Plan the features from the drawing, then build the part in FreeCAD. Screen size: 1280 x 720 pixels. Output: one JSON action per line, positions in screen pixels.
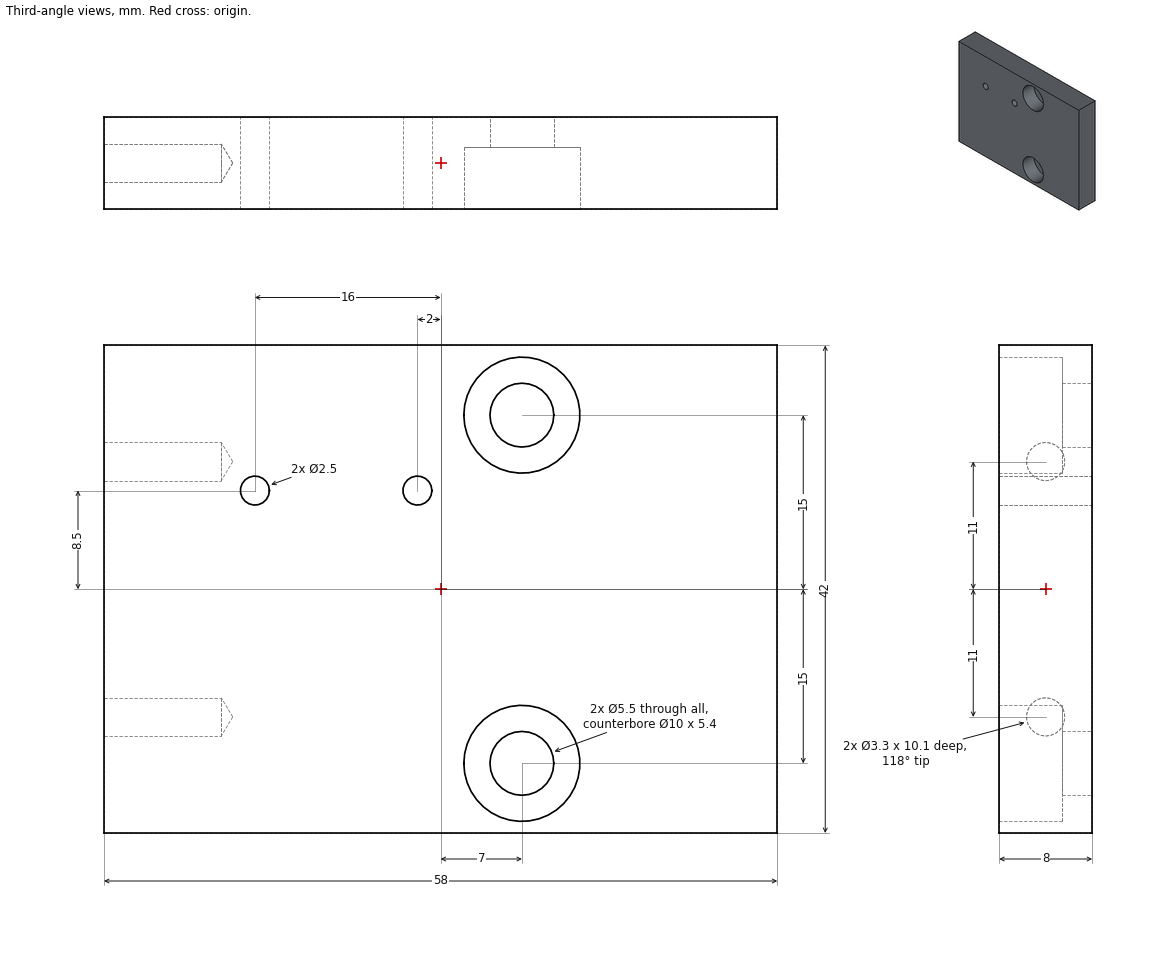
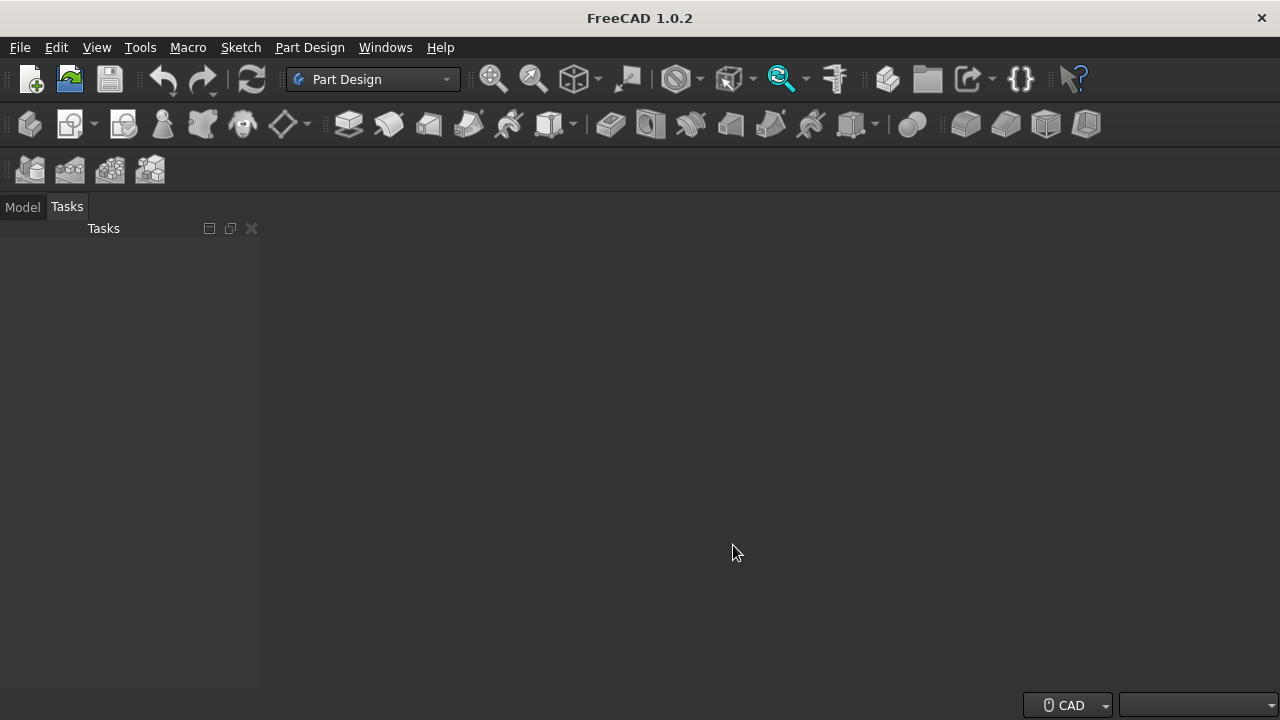
{"action": "left_click", "coordinate": [30, 80]}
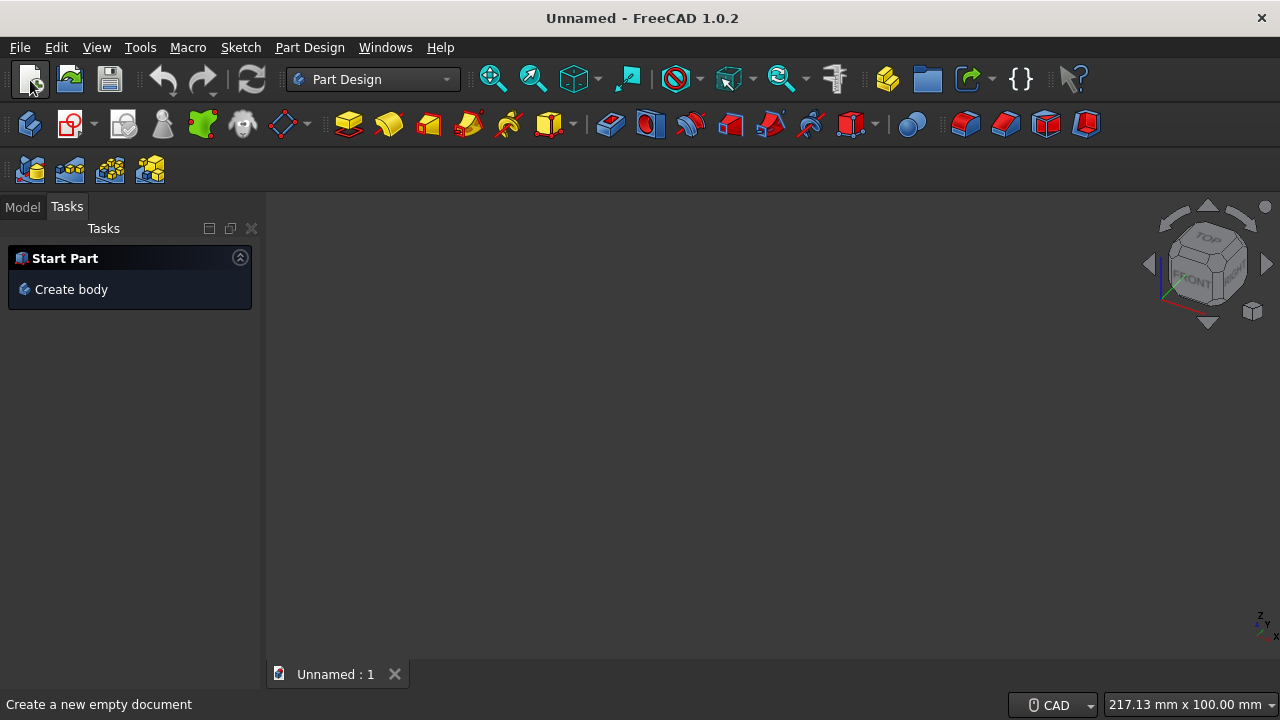
{"action": "left_click", "coordinate": [70, 124]}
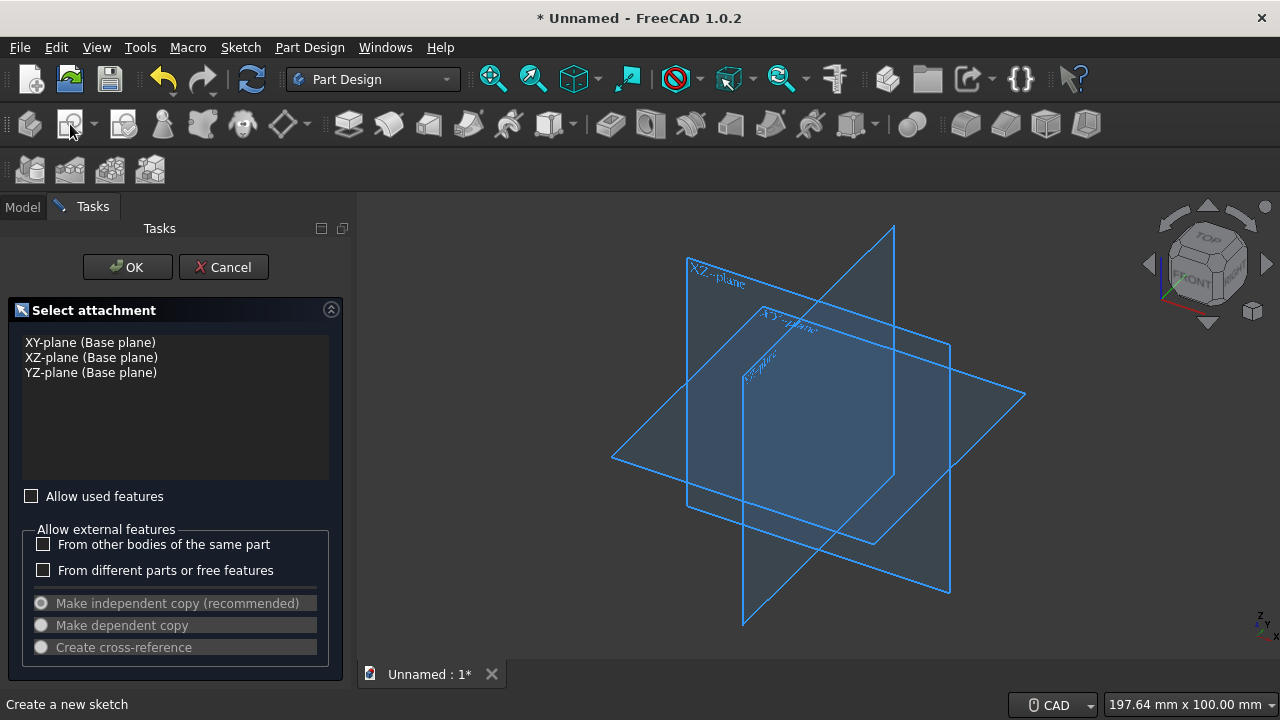
{"action": "left_click", "coordinate": [82, 358]}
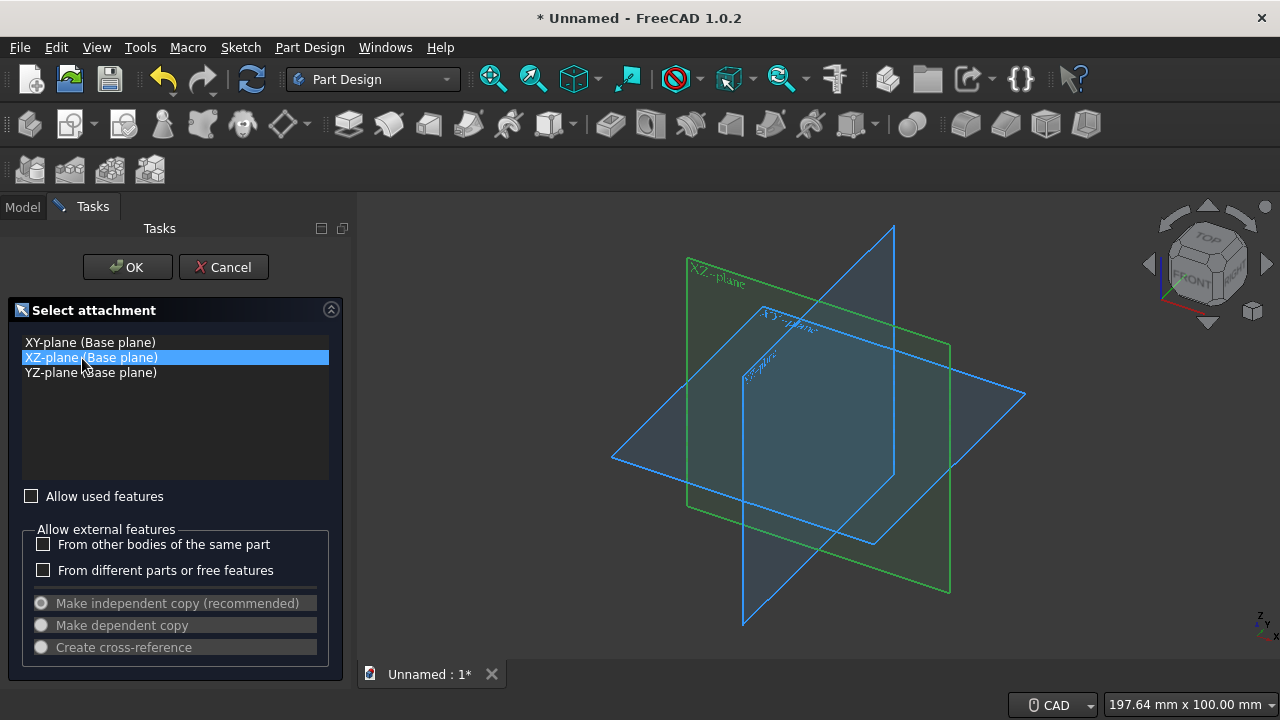
{"action": "left_click", "coordinate": [128, 267]}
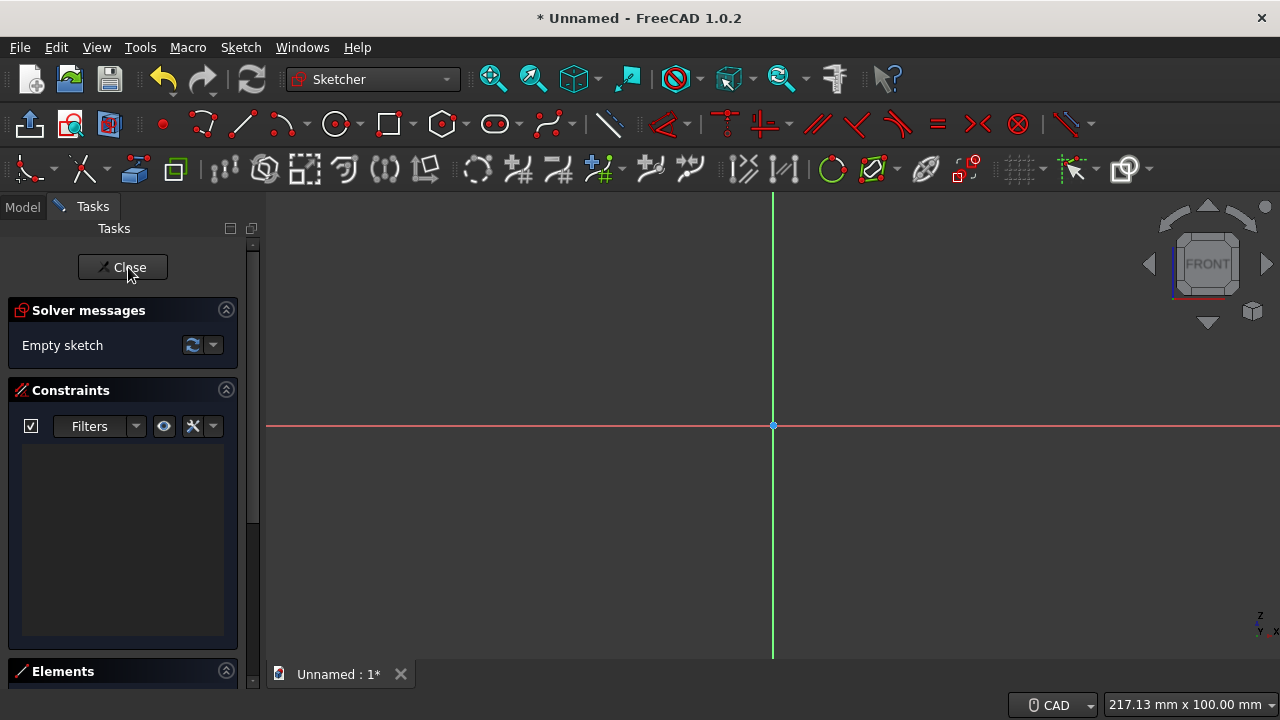
{"action": "scroll", "coordinate": [912, 425], "scroll_direction": "up", "scroll_amount": 2}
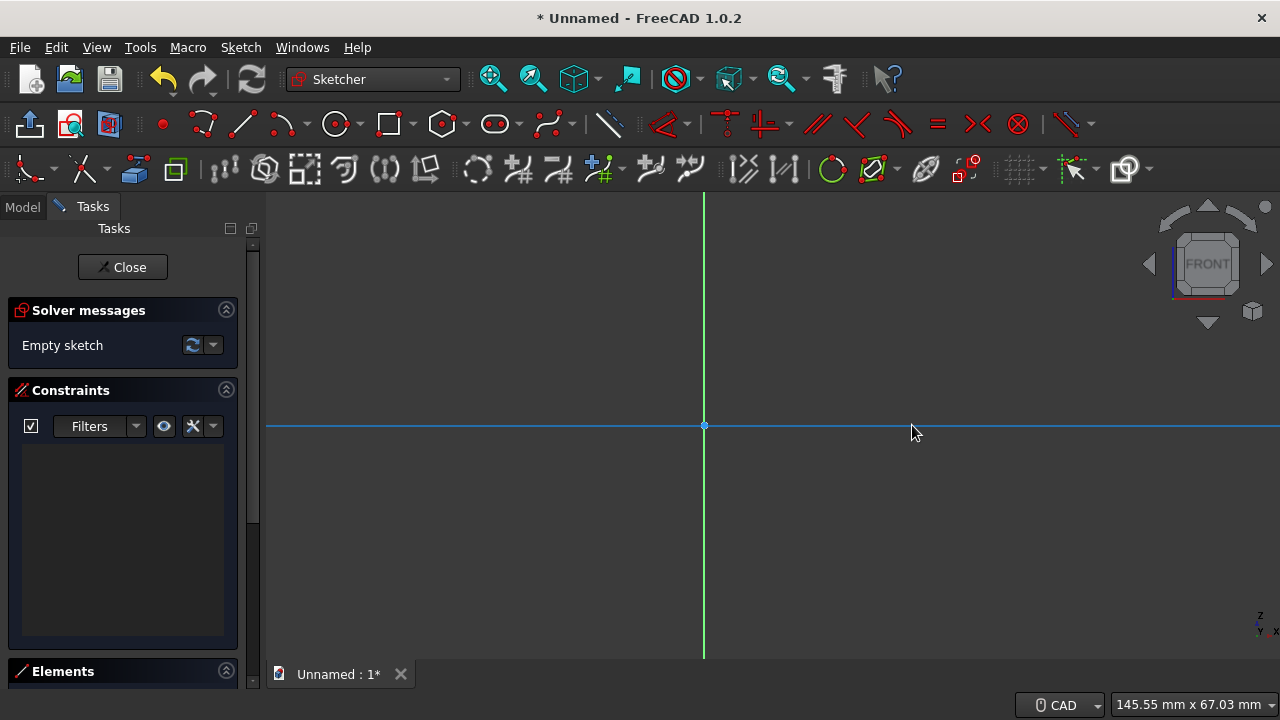
{"action": "key", "text": "g v"}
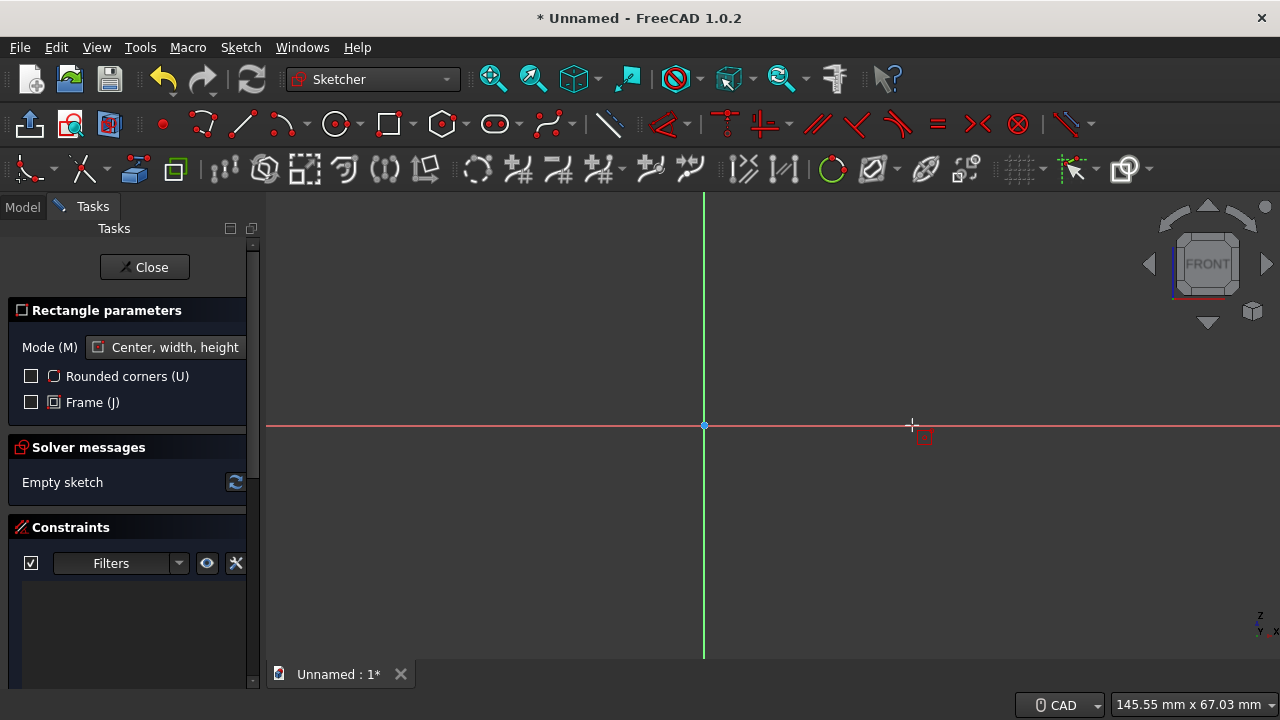
{"action": "left_click", "coordinate": [704, 426]}
{"action": "left_click", "coordinate": [906, 279]}
{"action": "key", "text": "Escape"}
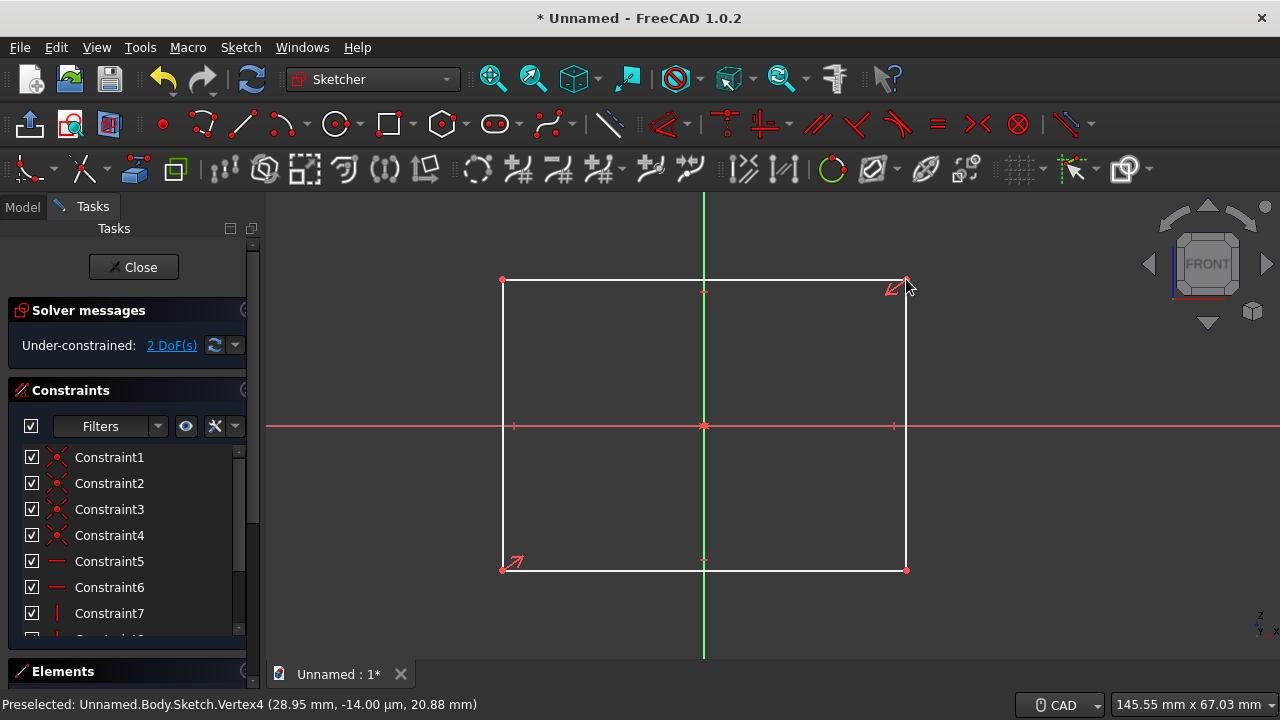
{"action": "left_click", "coordinate": [664, 124]}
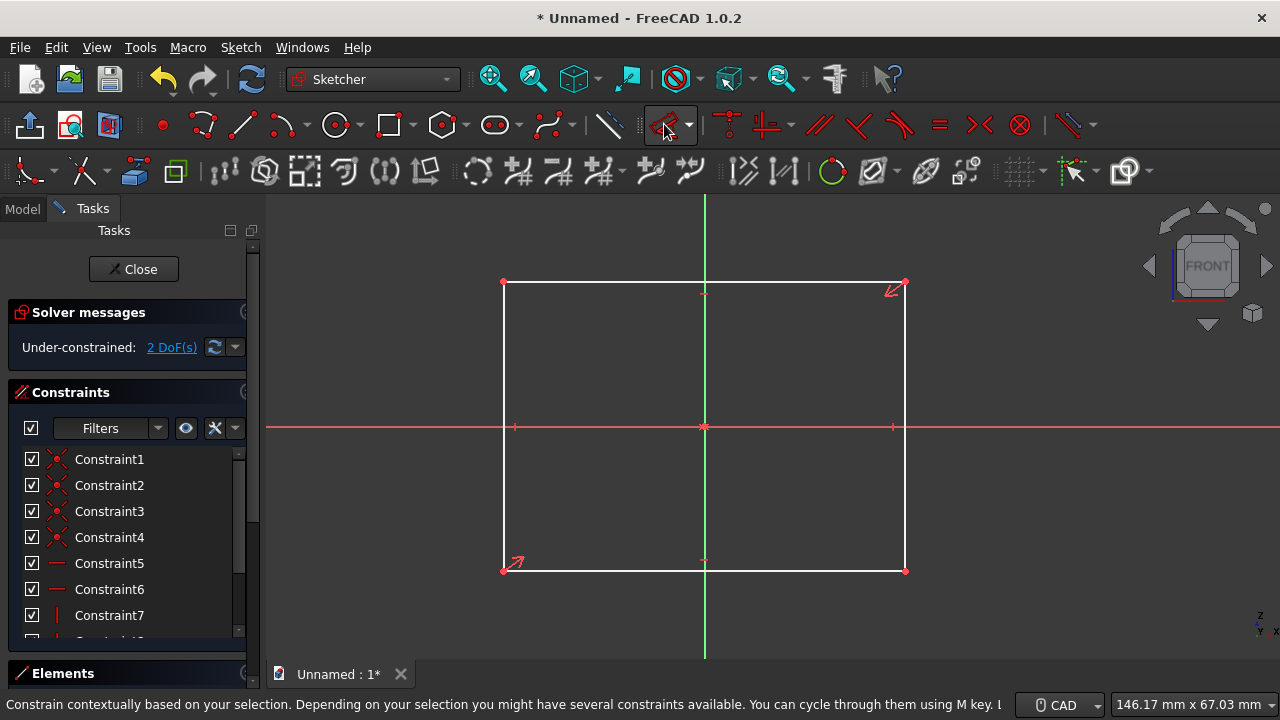
{"action": "left_click", "coordinate": [624, 571]}
{"action": "left_click", "coordinate": [612, 605]}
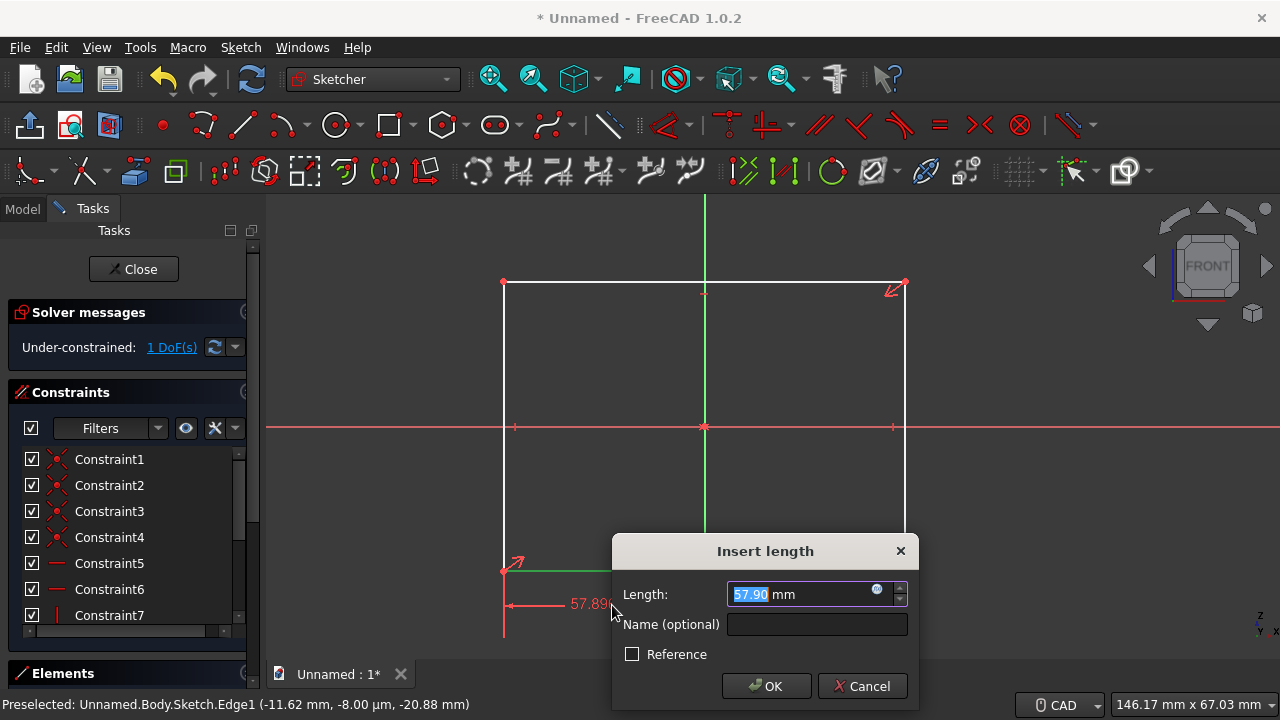
{"action": "type", "text": "58"}
{"action": "key", "text": "Return"}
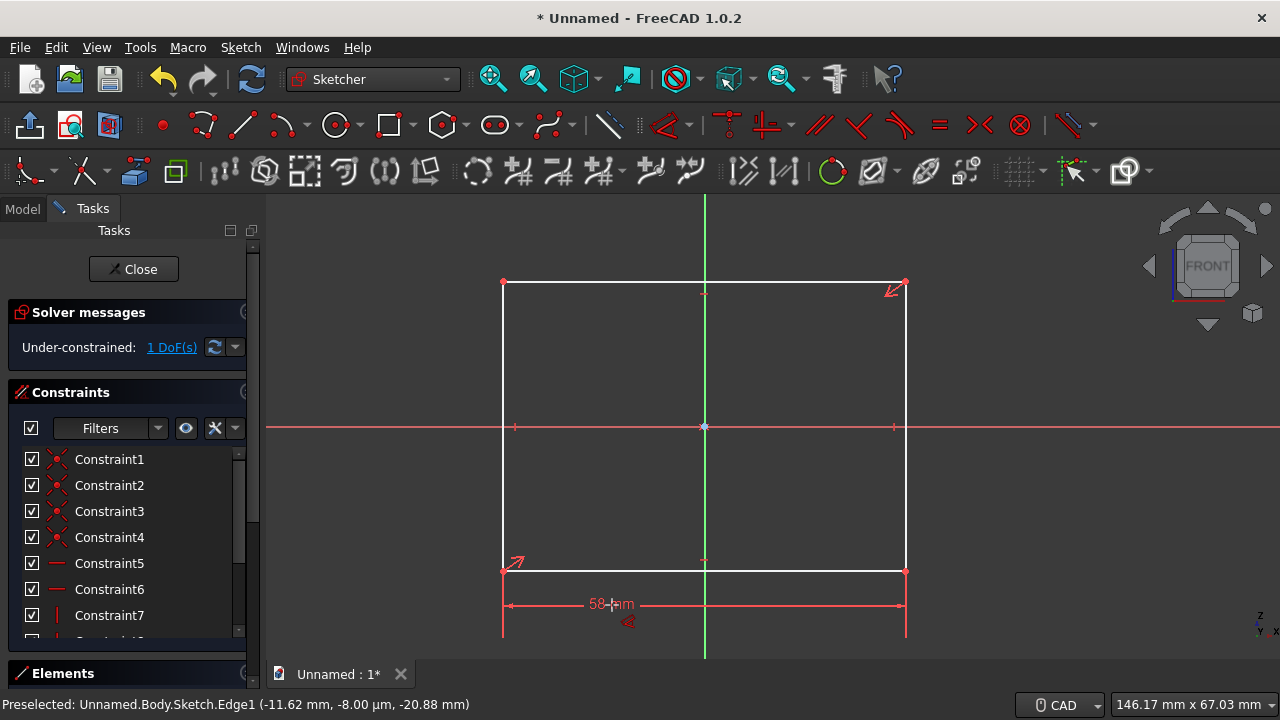
{"action": "left_click", "coordinate": [906, 484]}
{"action": "left_click", "coordinate": [940, 360]}